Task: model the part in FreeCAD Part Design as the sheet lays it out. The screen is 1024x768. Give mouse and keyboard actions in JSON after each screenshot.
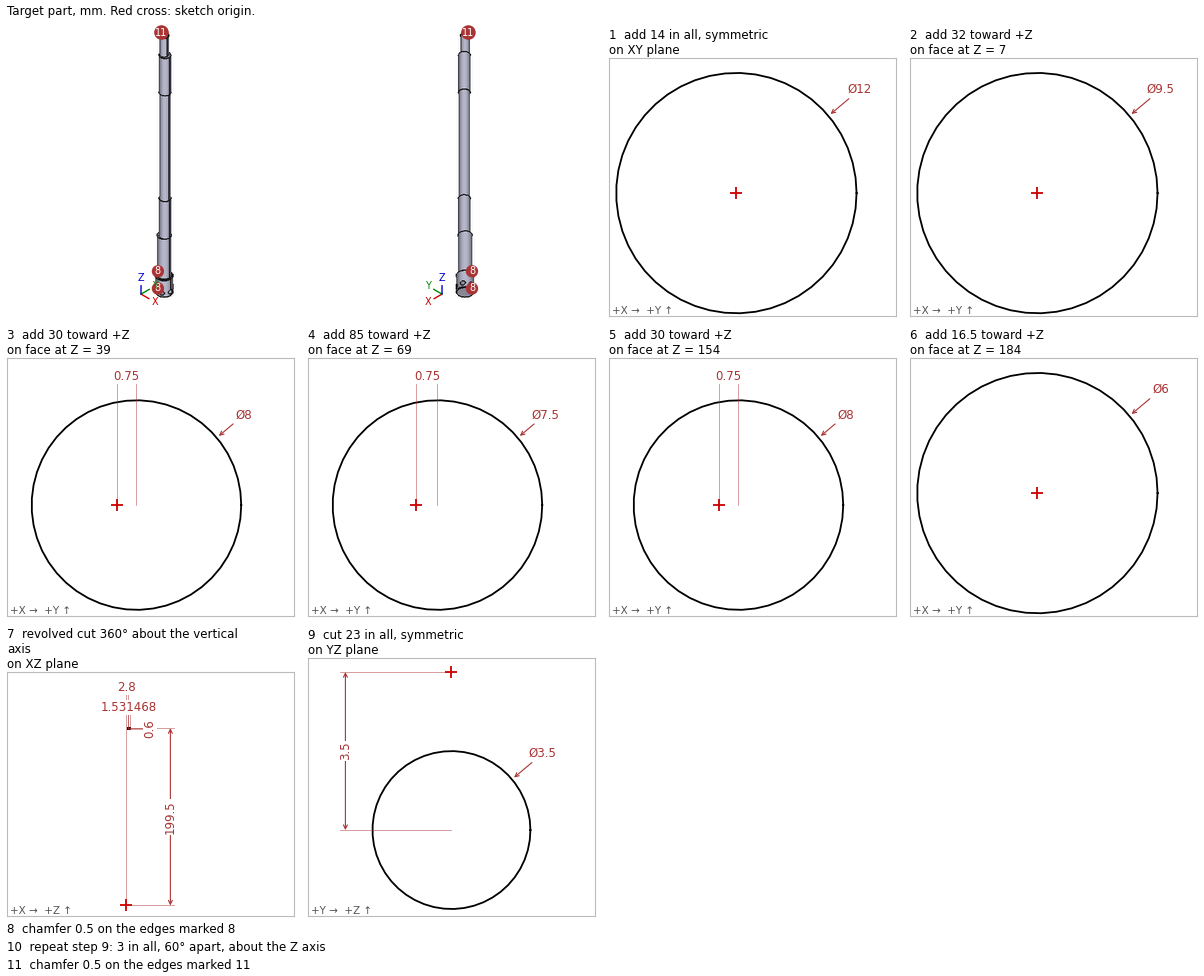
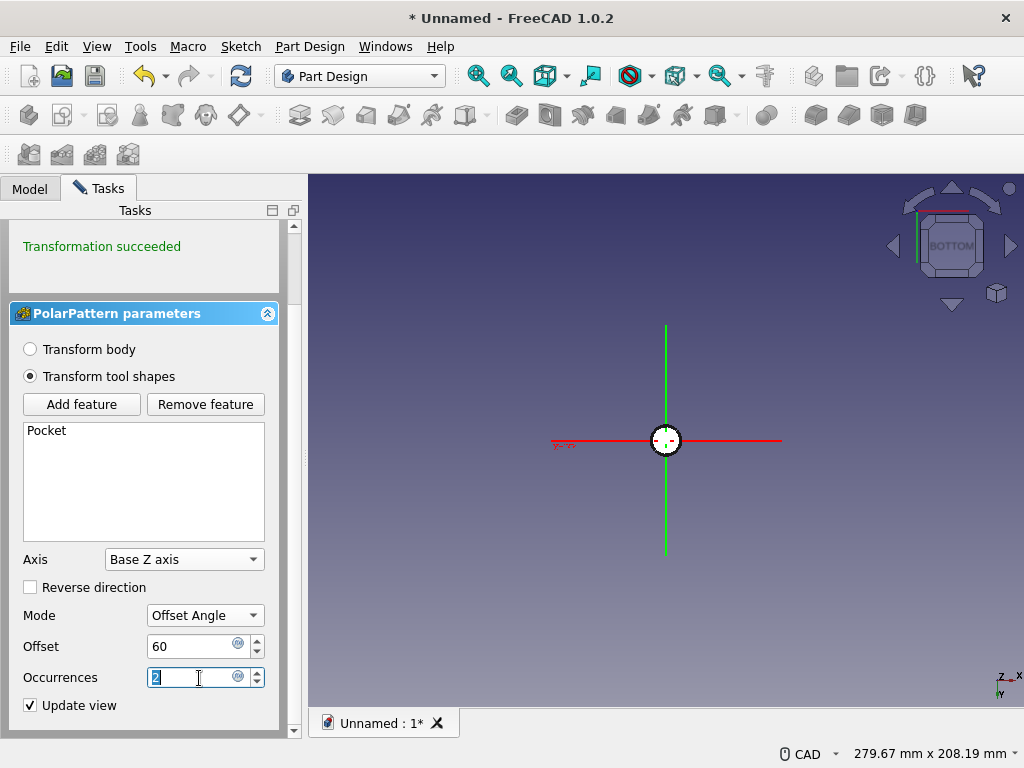
{"action": "type", "text": "3"}
{"action": "key", "text": "Tab"}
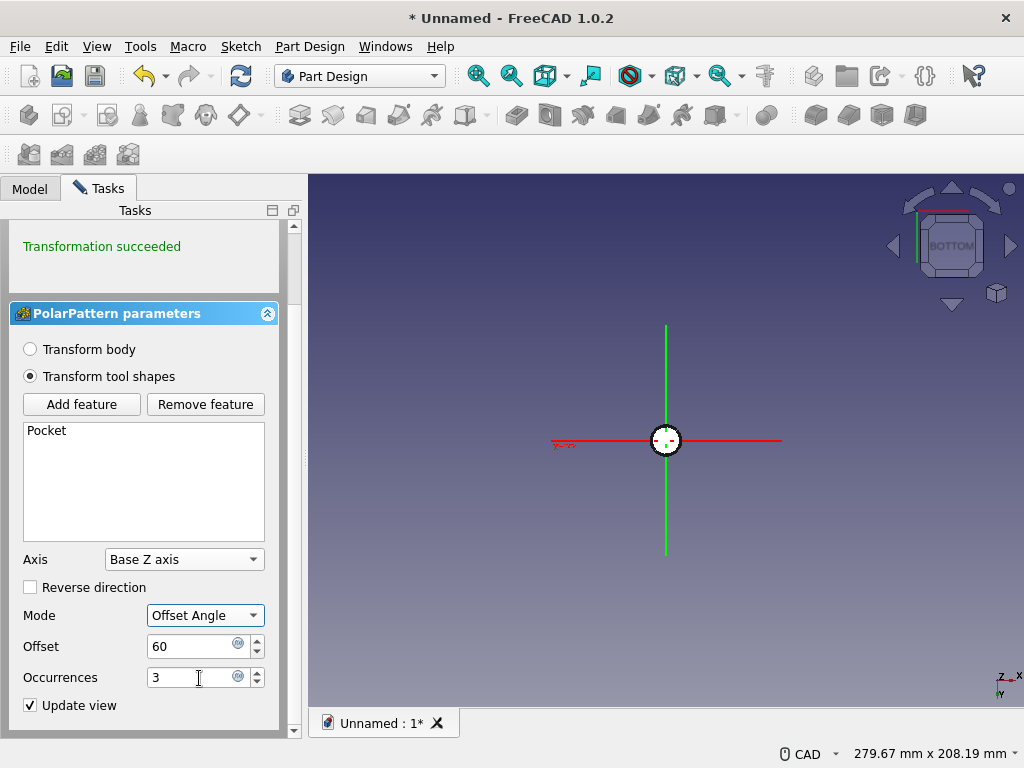
{"action": "scroll", "coordinate": [294, 479], "scroll_direction": "up", "scroll_amount": 3}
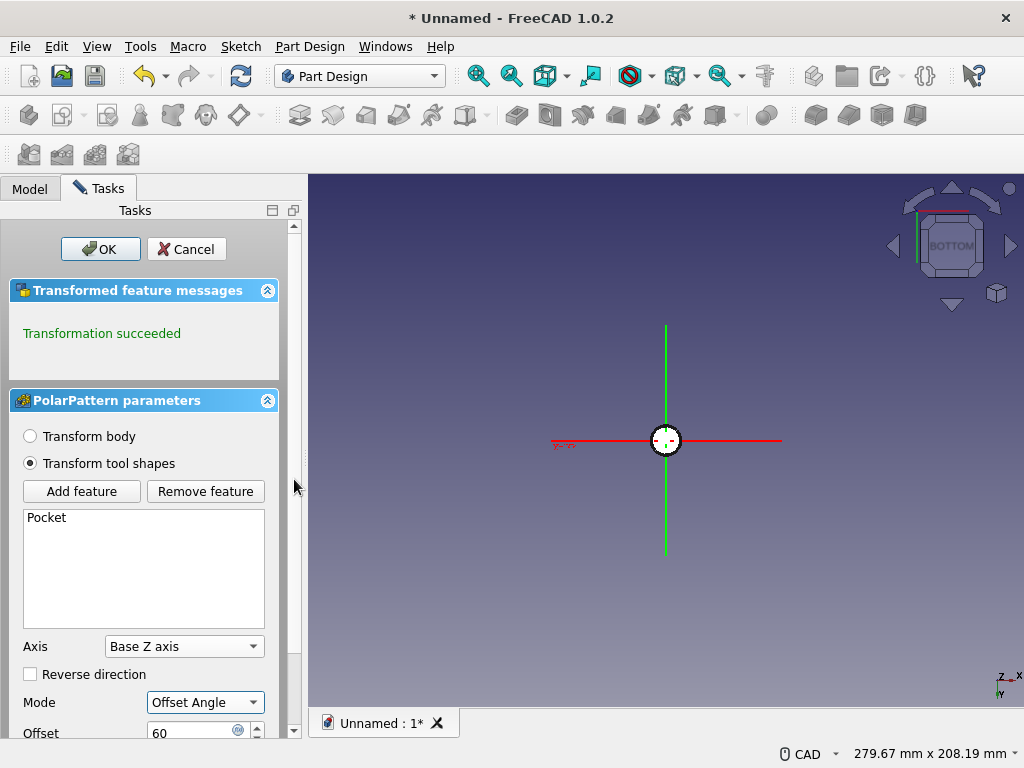
{"action": "left_click", "coordinate": [101, 249]}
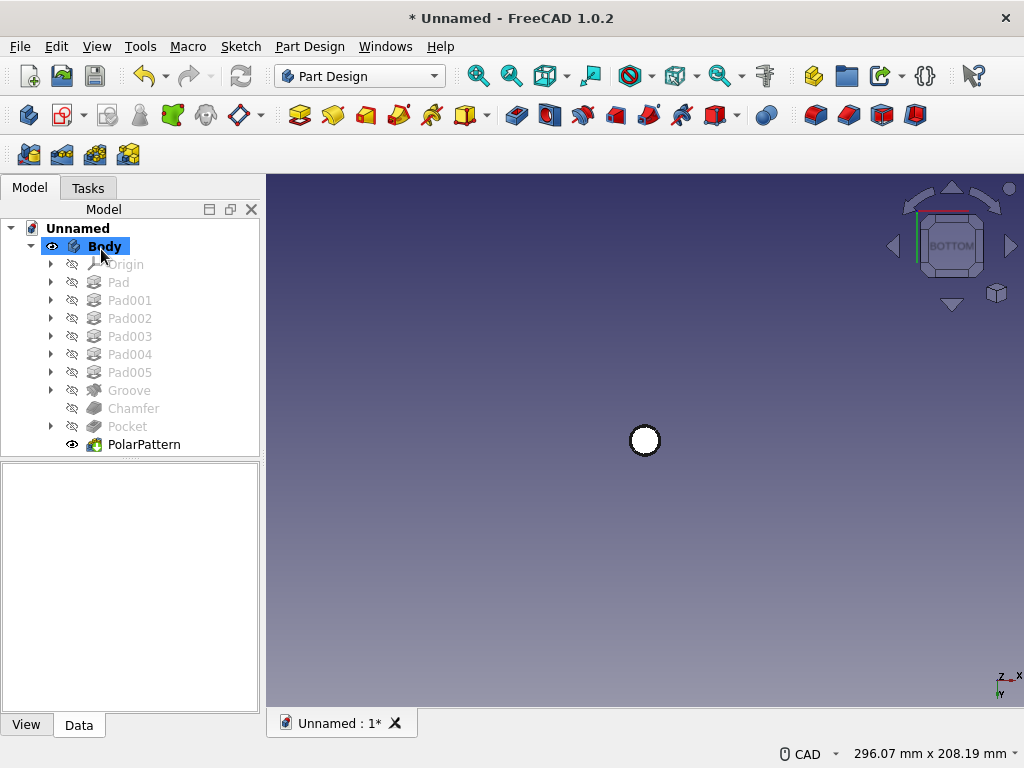
{"action": "key", "text": "v f"}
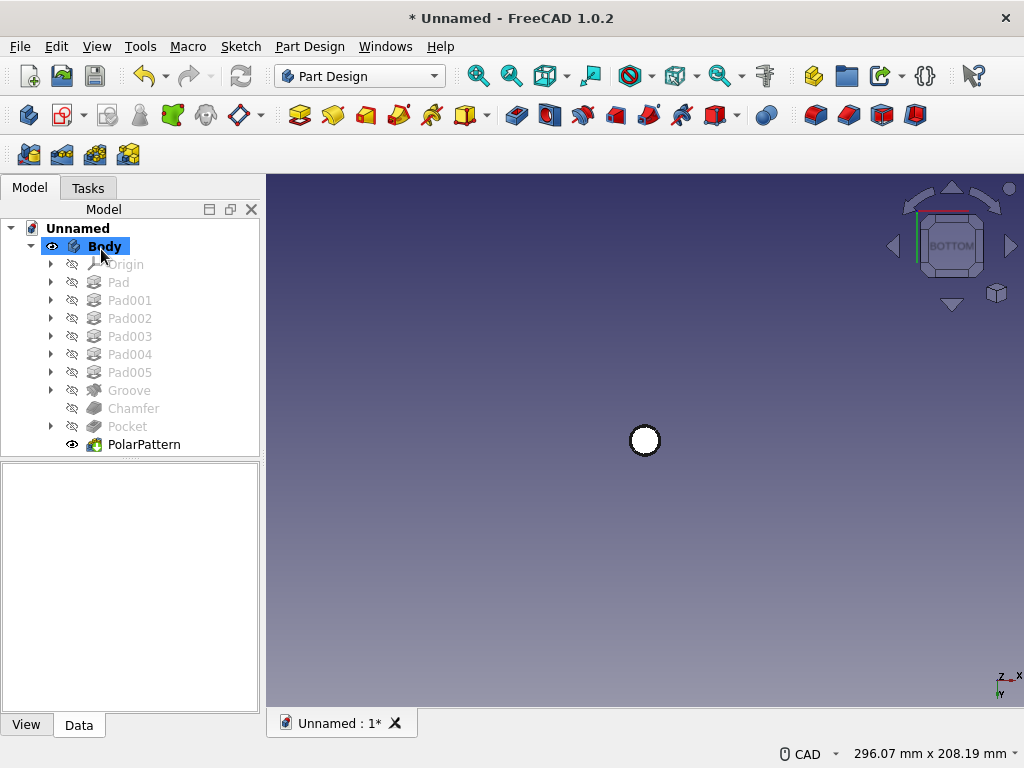
{"action": "key", "text": "0"}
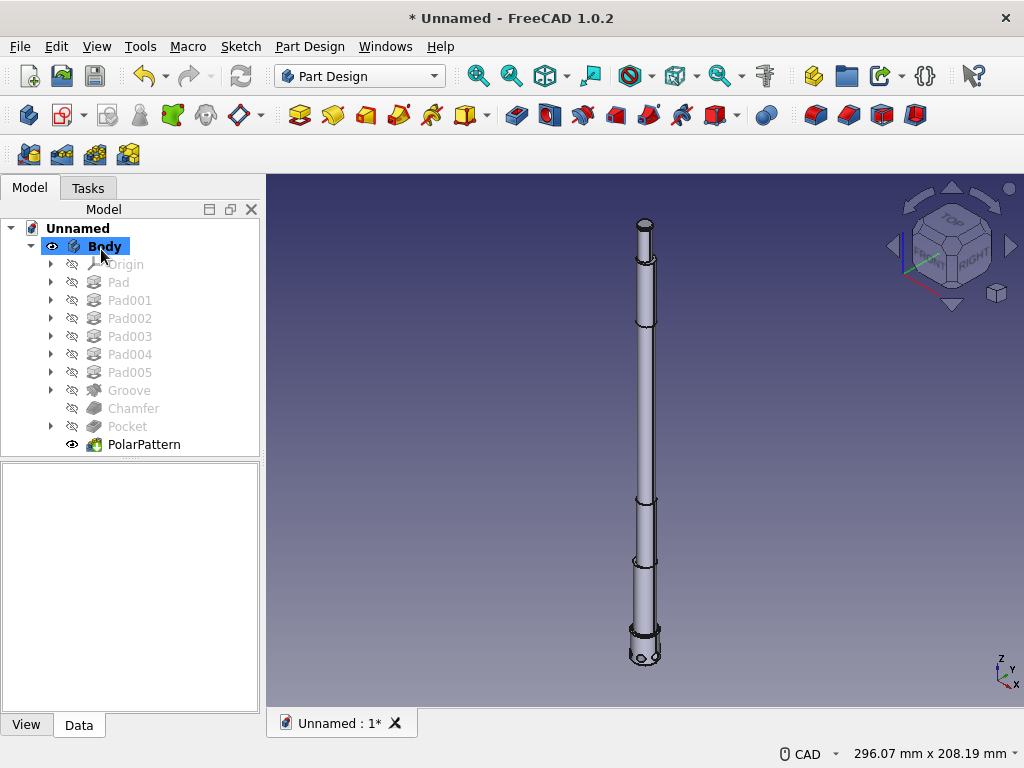
{"action": "left_click", "coordinate": [640, 219]}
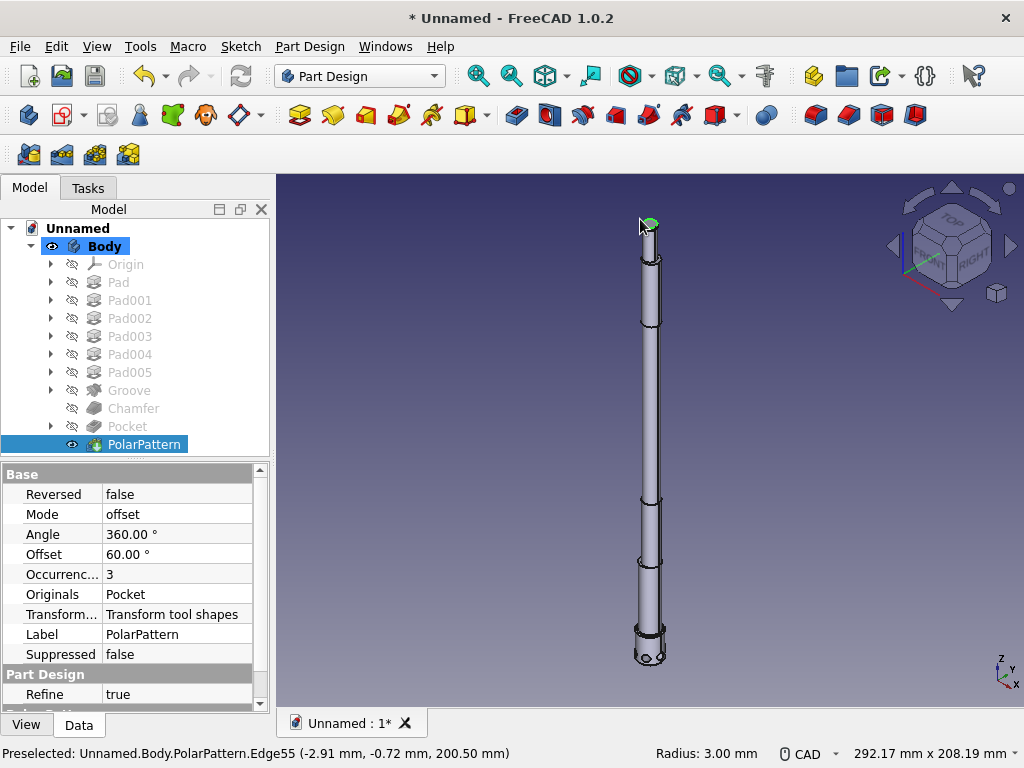
{"action": "left_click", "coordinate": [849, 116]}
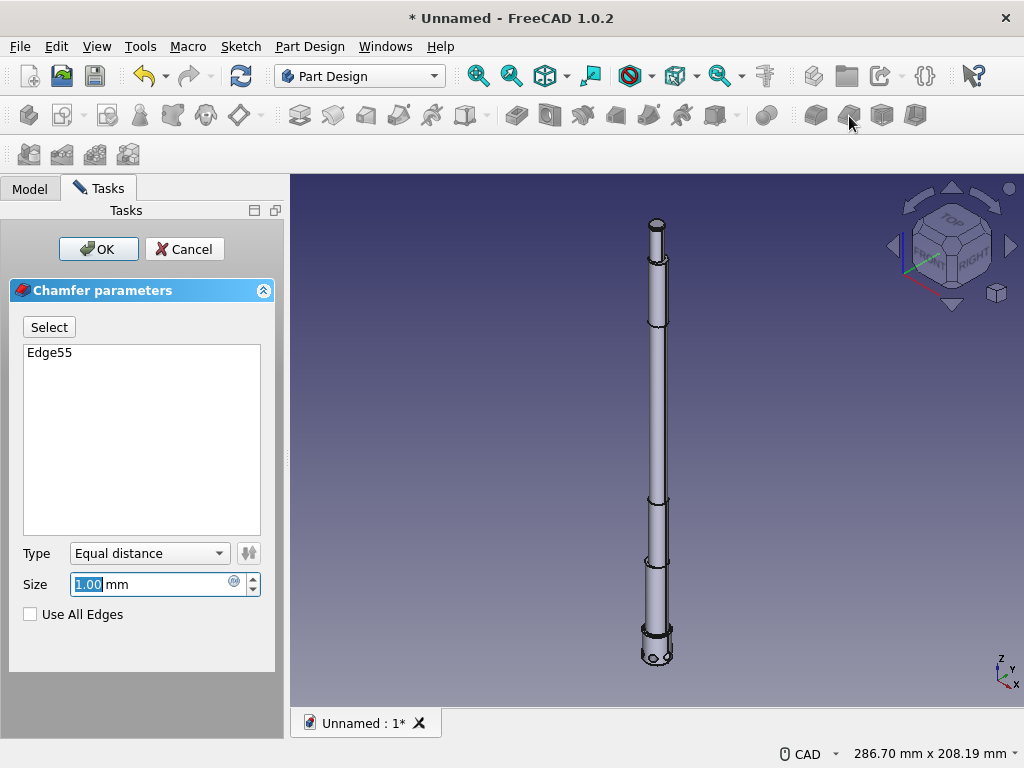
{"action": "type", "text": "0.5"}
{"action": "key", "text": "Tab"}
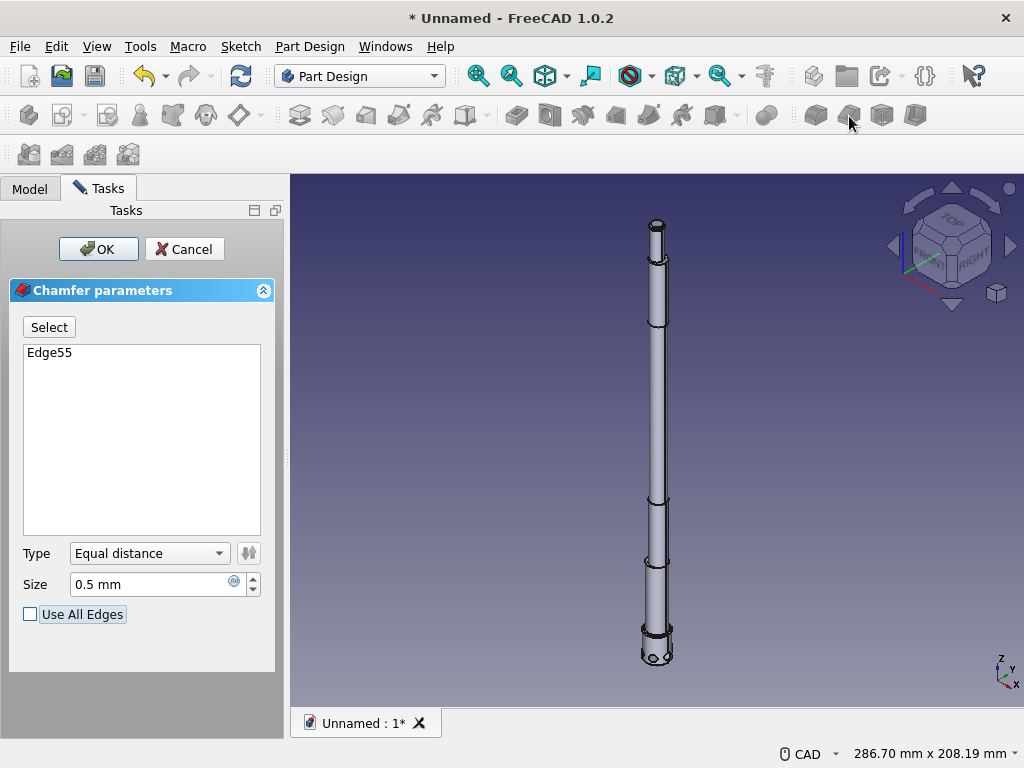
{"action": "left_click", "coordinate": [99, 249]}